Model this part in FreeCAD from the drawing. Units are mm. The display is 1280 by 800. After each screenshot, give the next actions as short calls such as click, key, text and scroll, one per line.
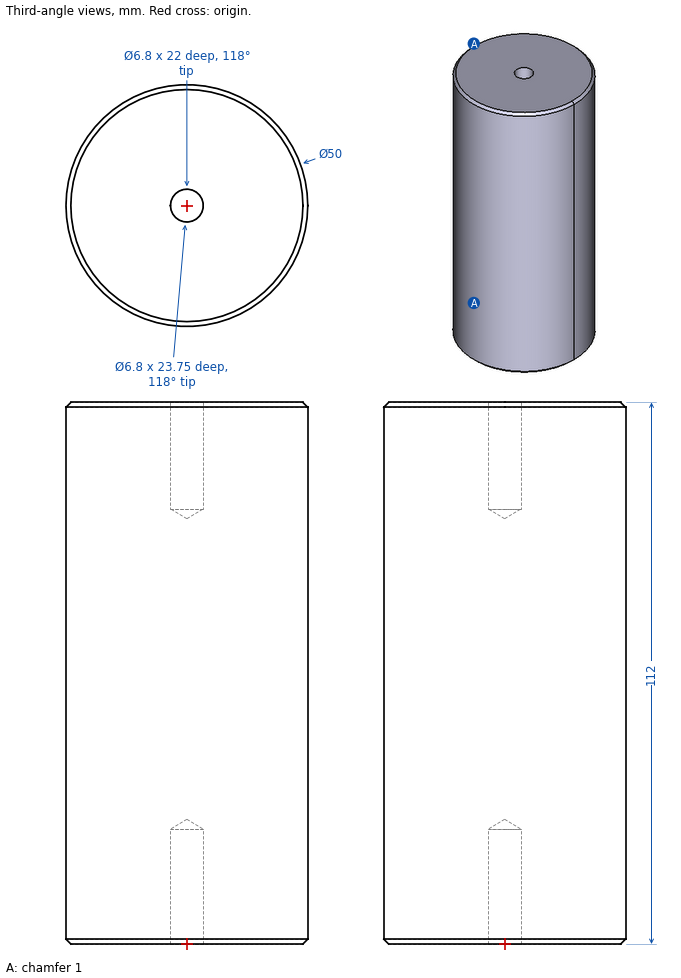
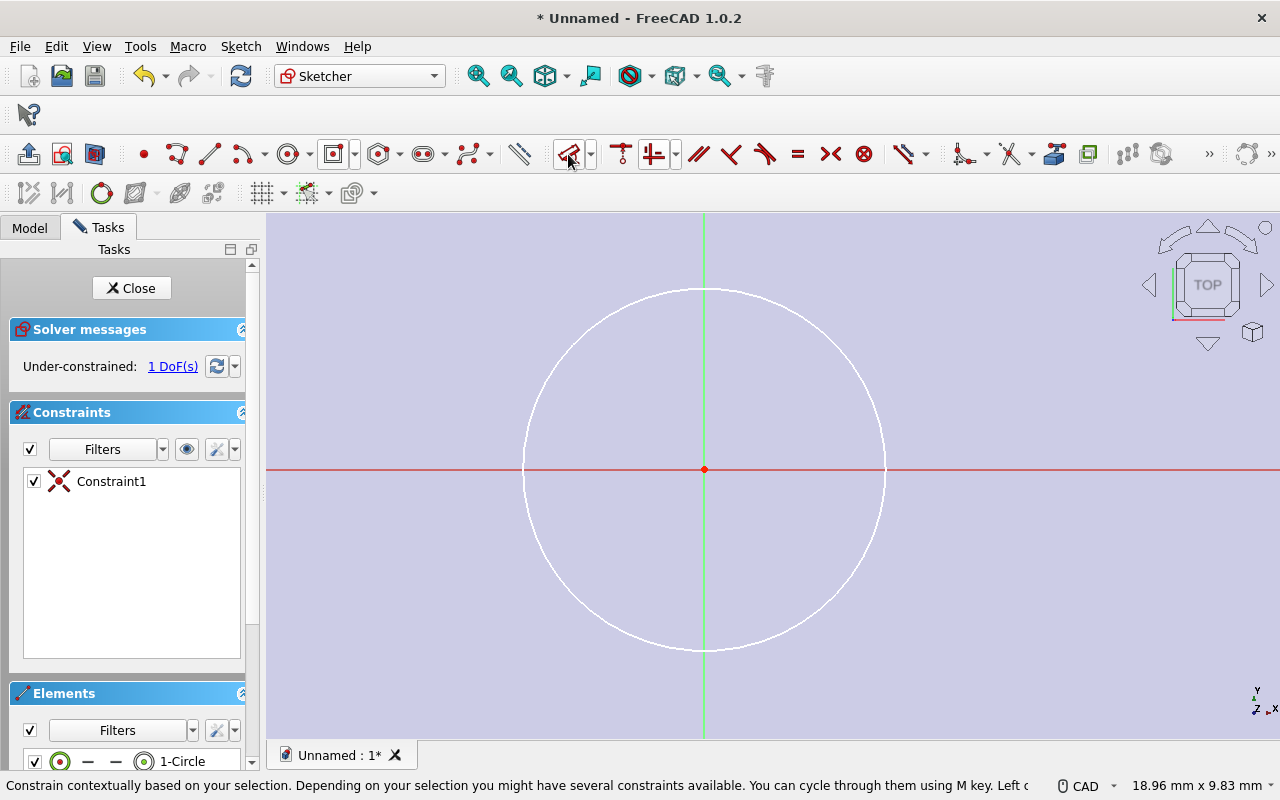
click(832, 341)
click(855, 318)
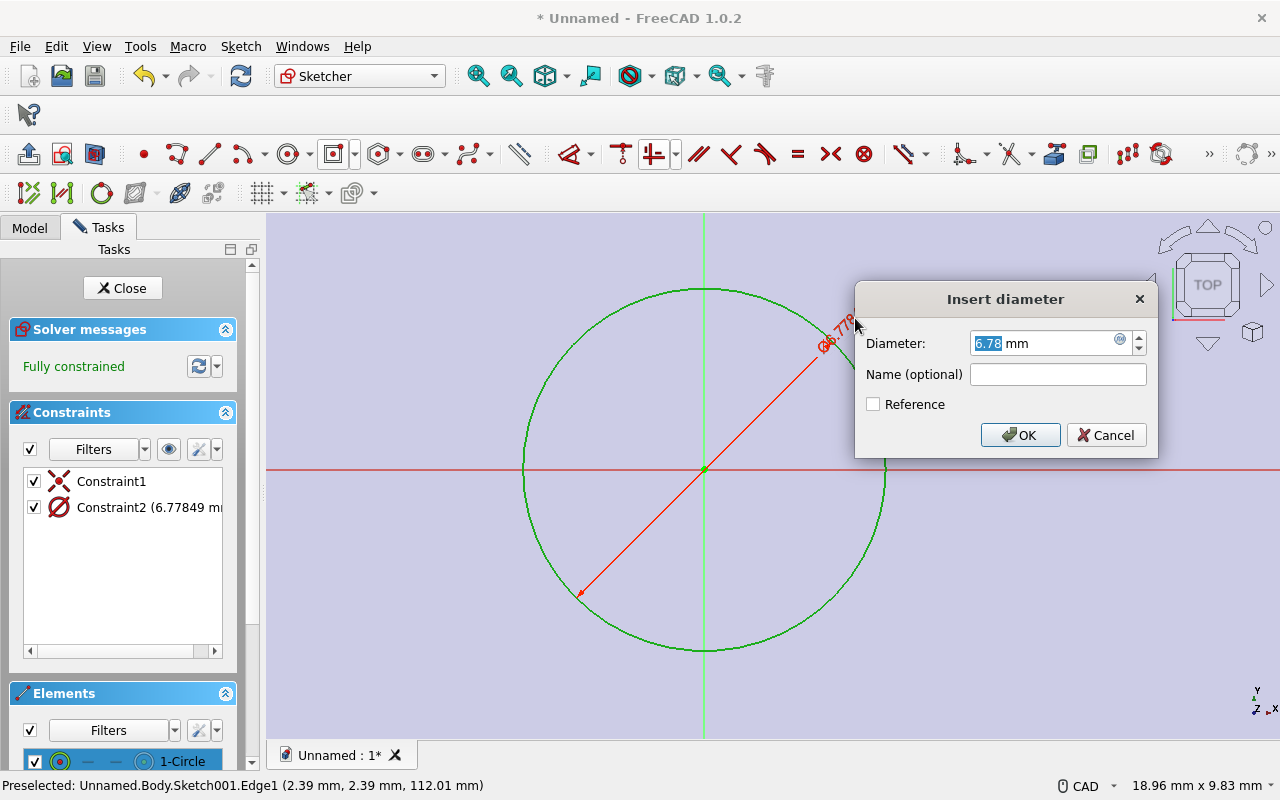
text(6.8)
key(Return)
key(Escape)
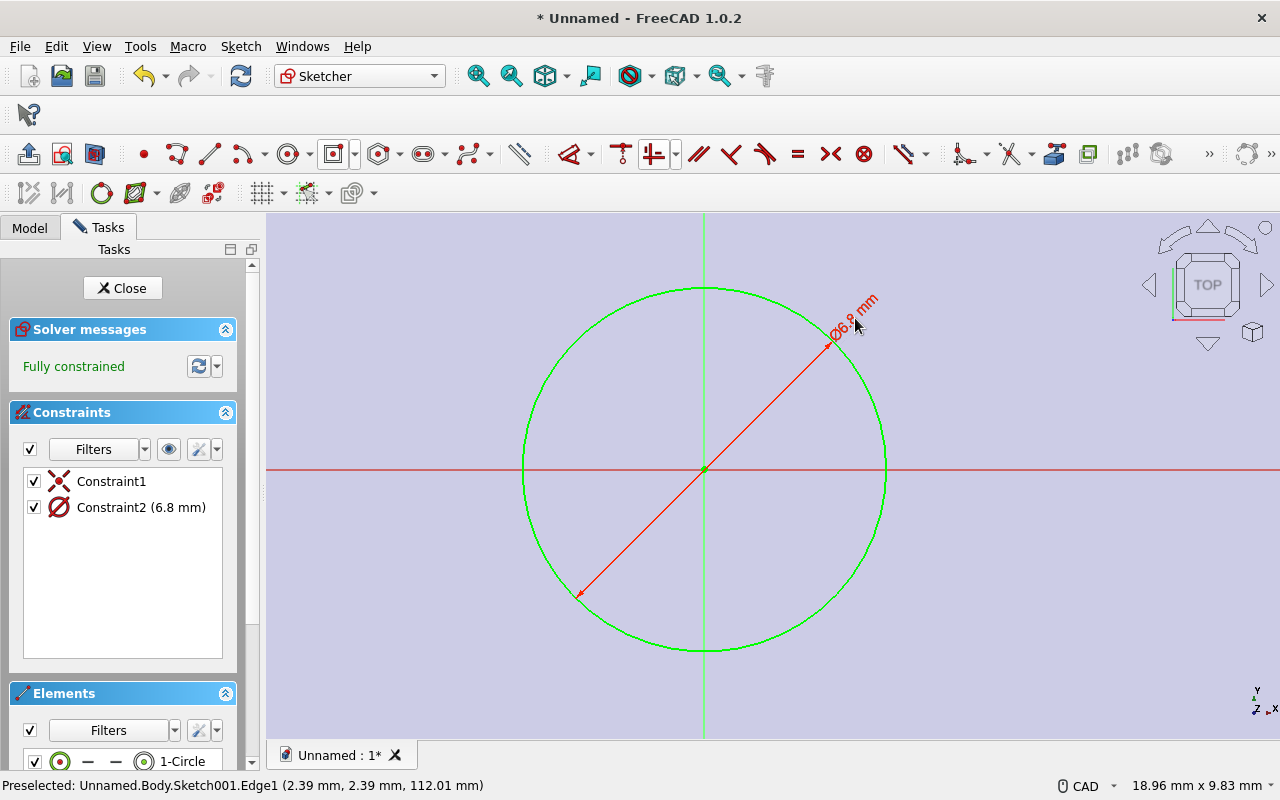
click(123, 288)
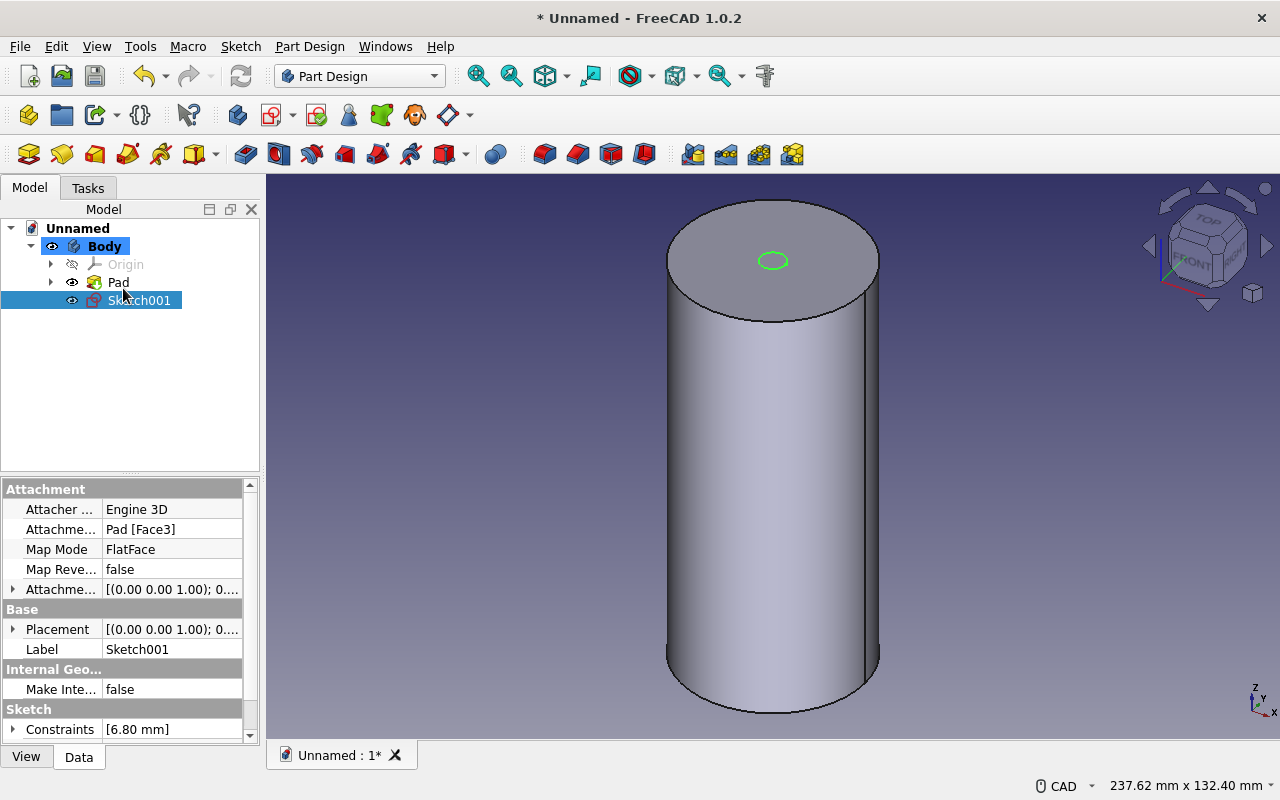
click(279, 154)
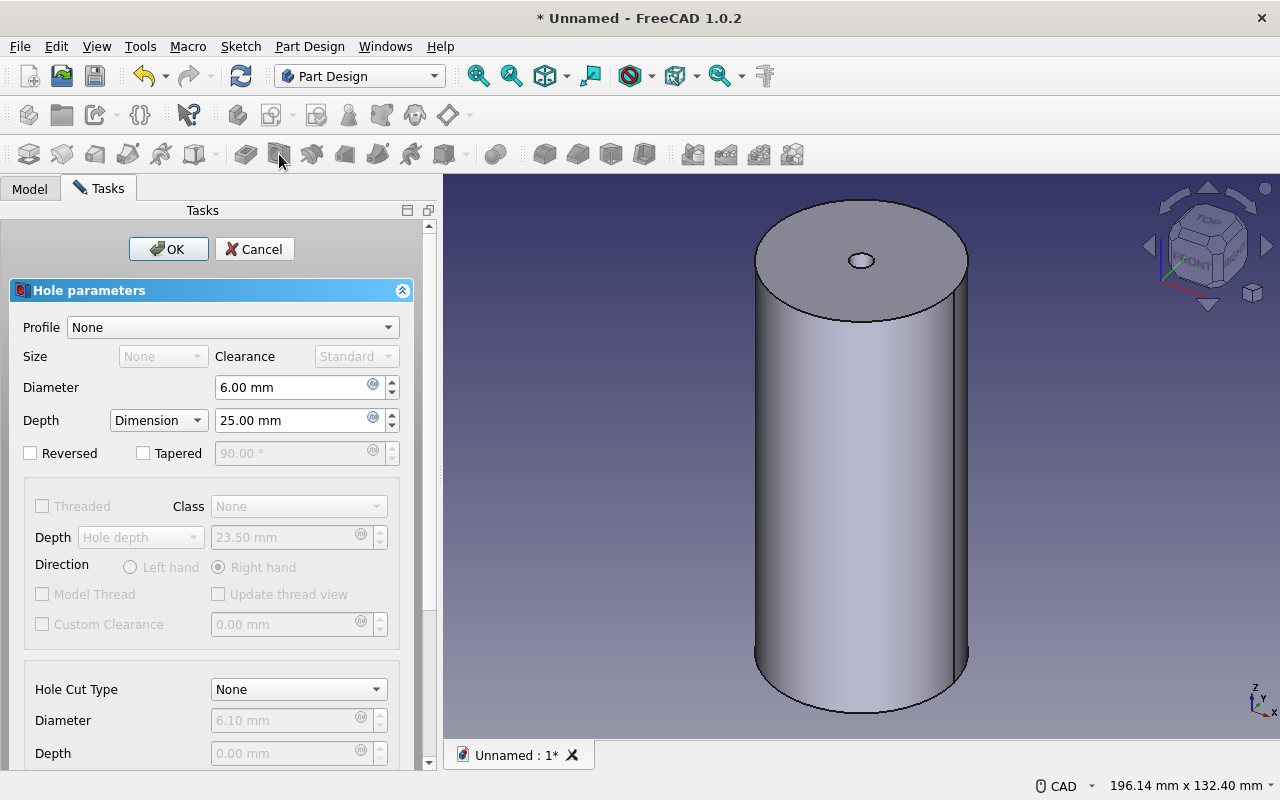
triple_click(300, 388)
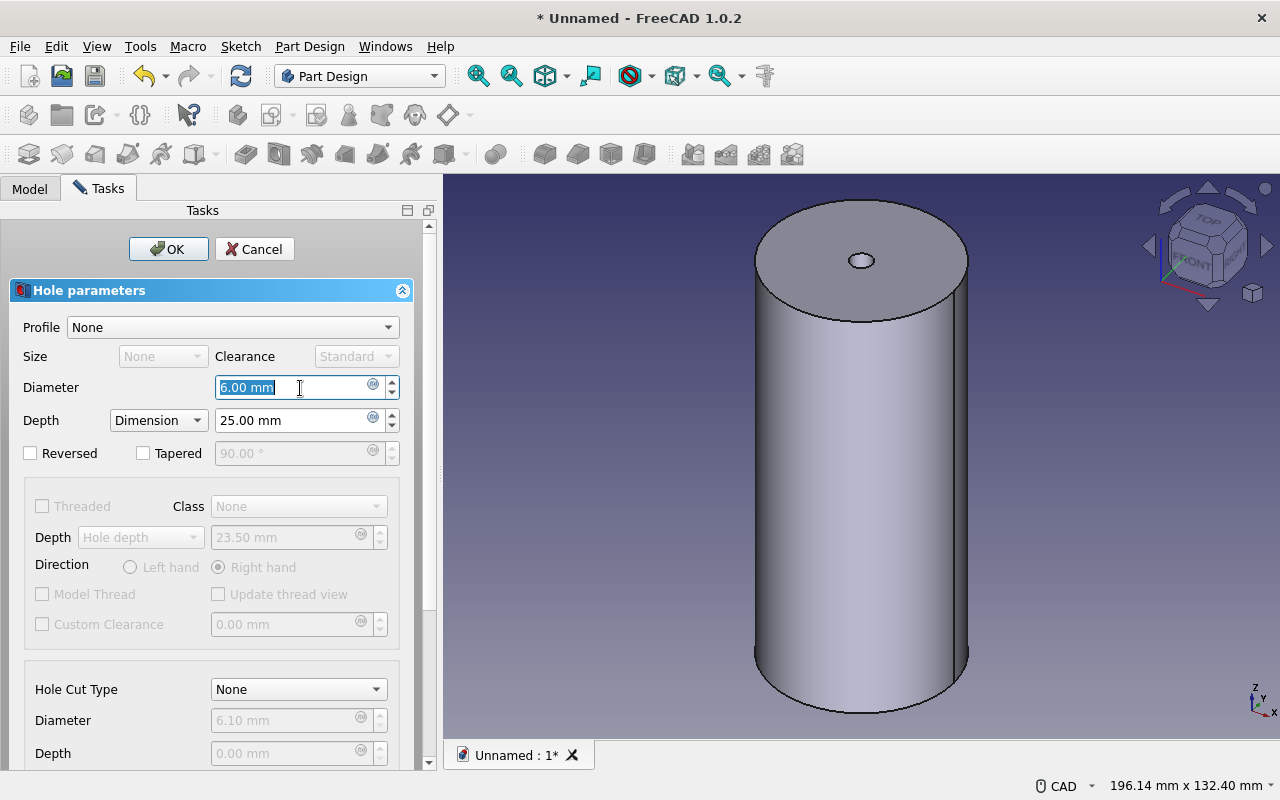
text(6.8)
key(Tab)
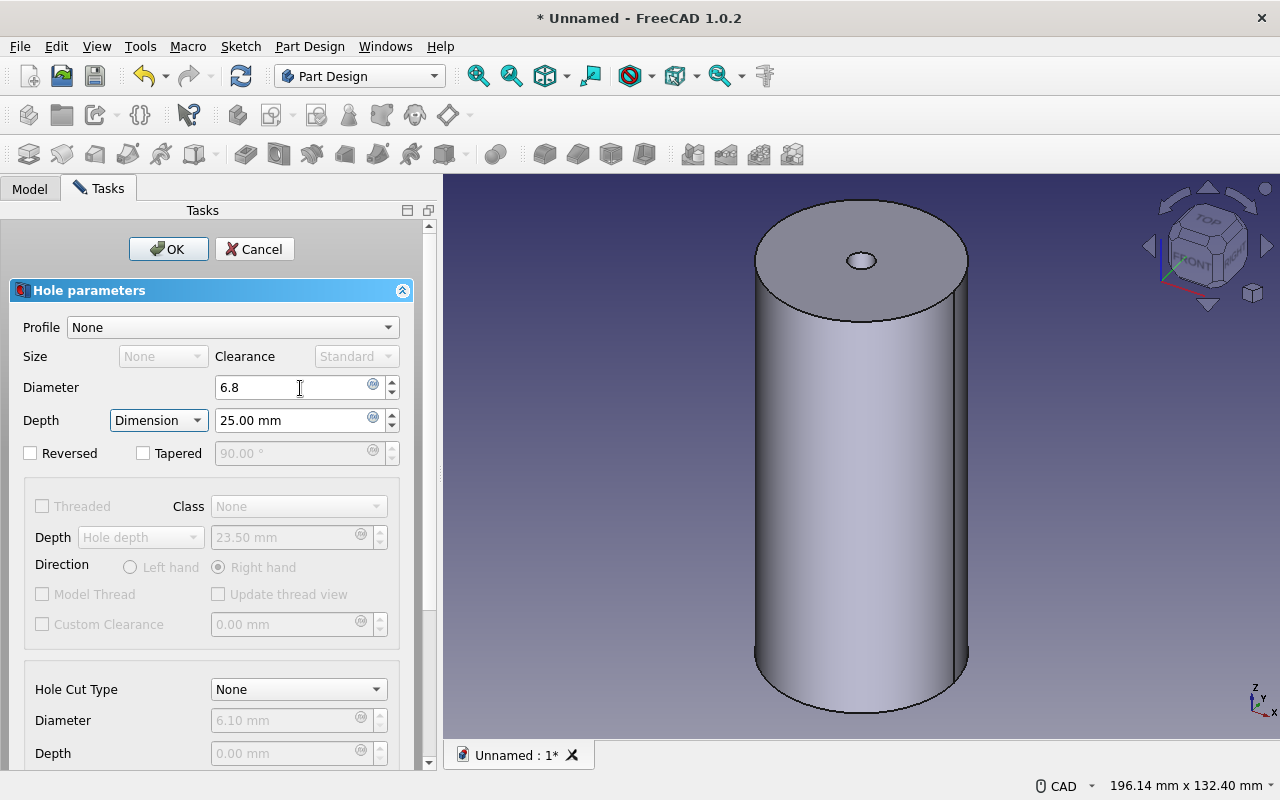
triple_click(300, 420)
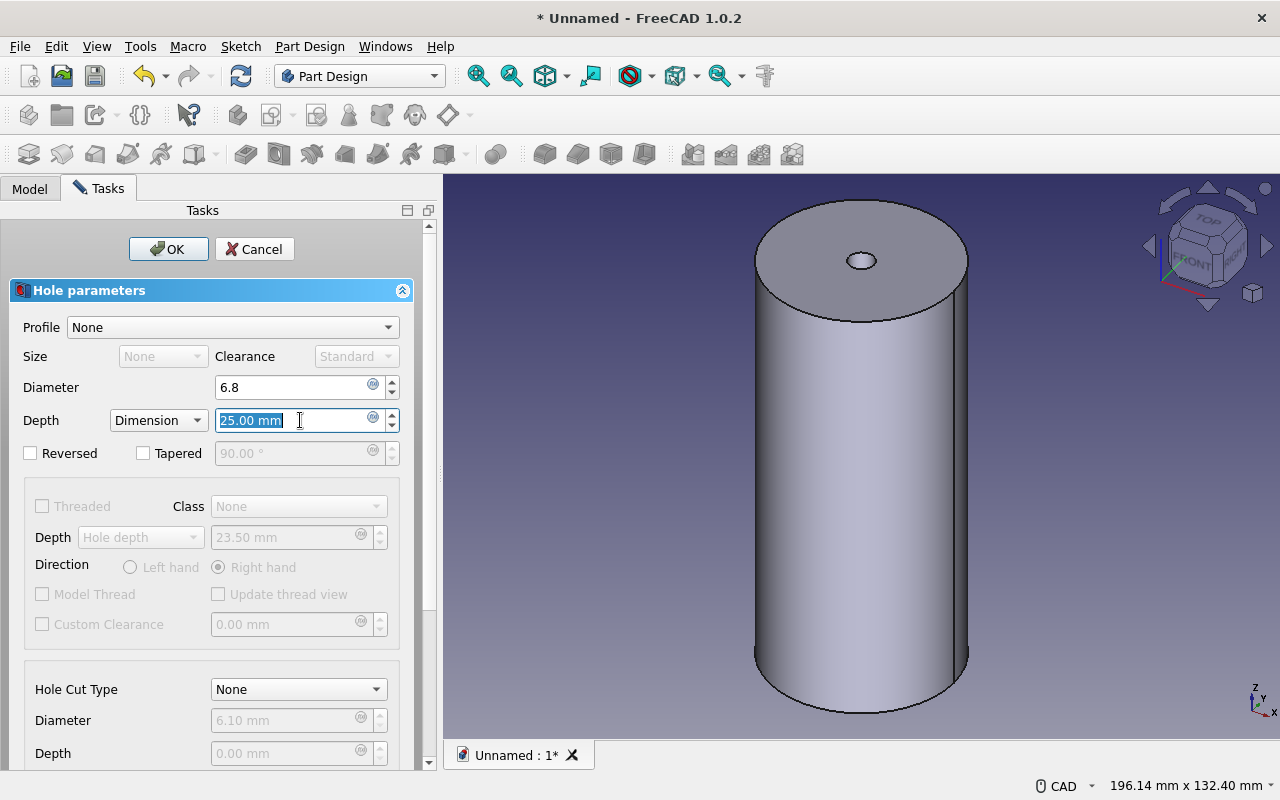
text(22)
key(Tab)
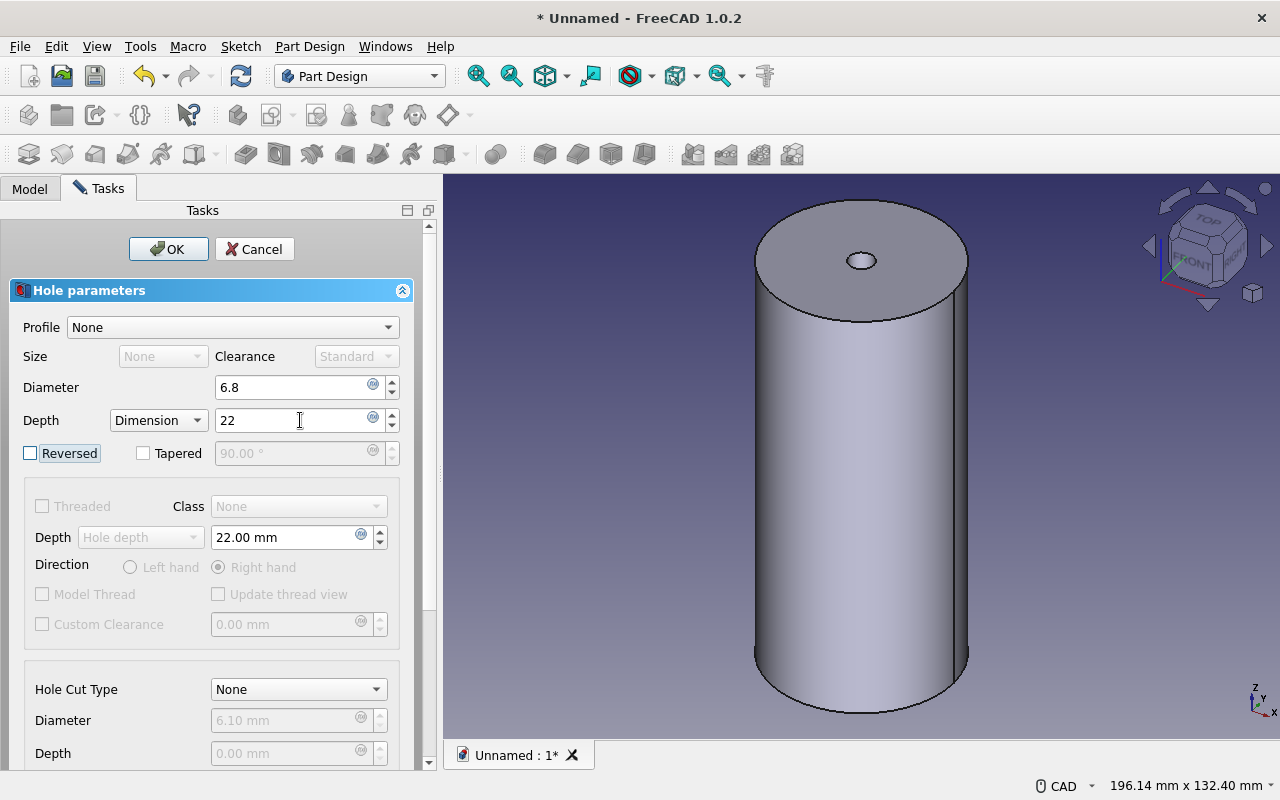
click(169, 249)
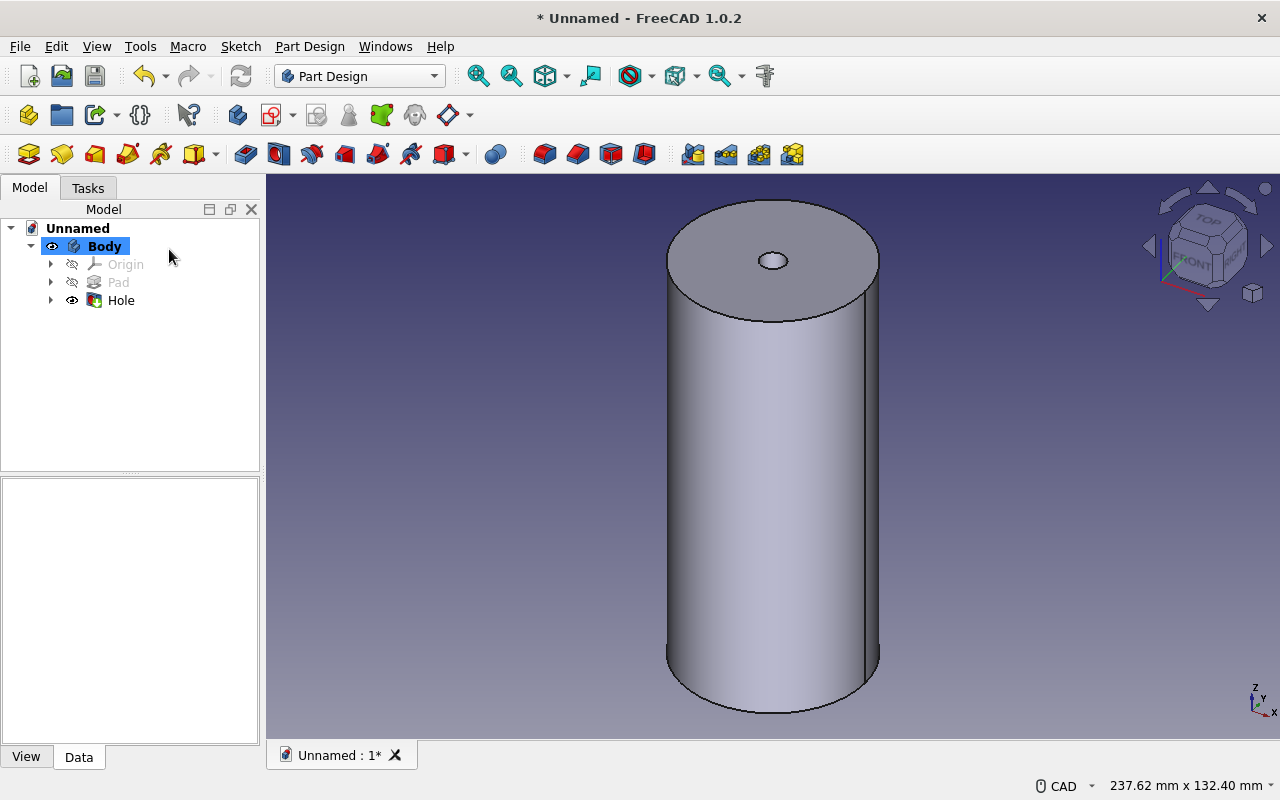
key(5)